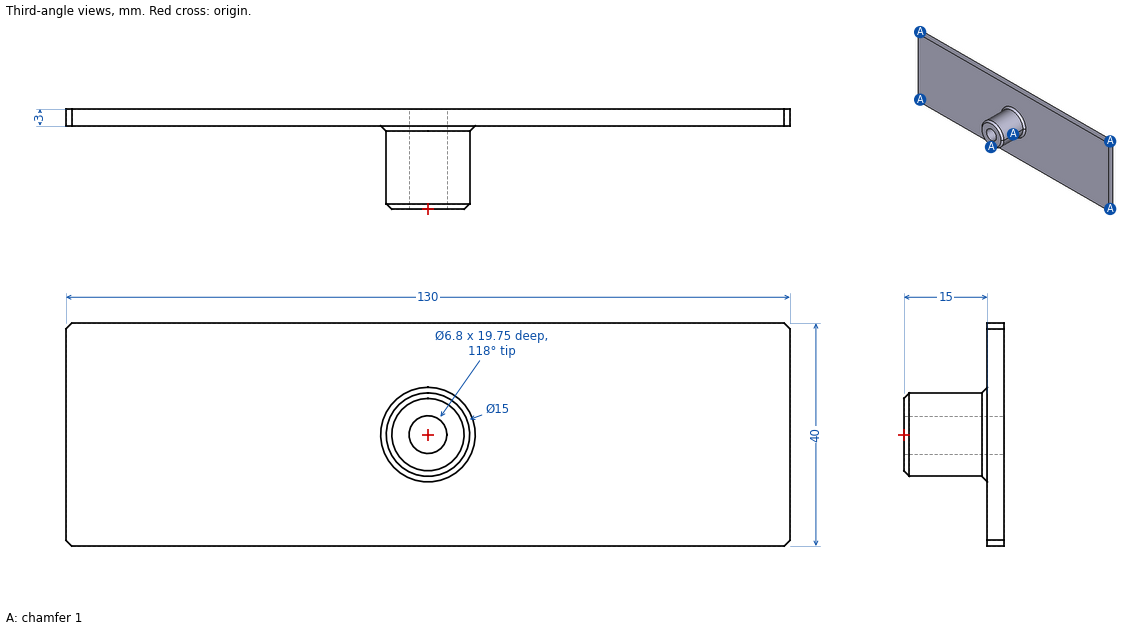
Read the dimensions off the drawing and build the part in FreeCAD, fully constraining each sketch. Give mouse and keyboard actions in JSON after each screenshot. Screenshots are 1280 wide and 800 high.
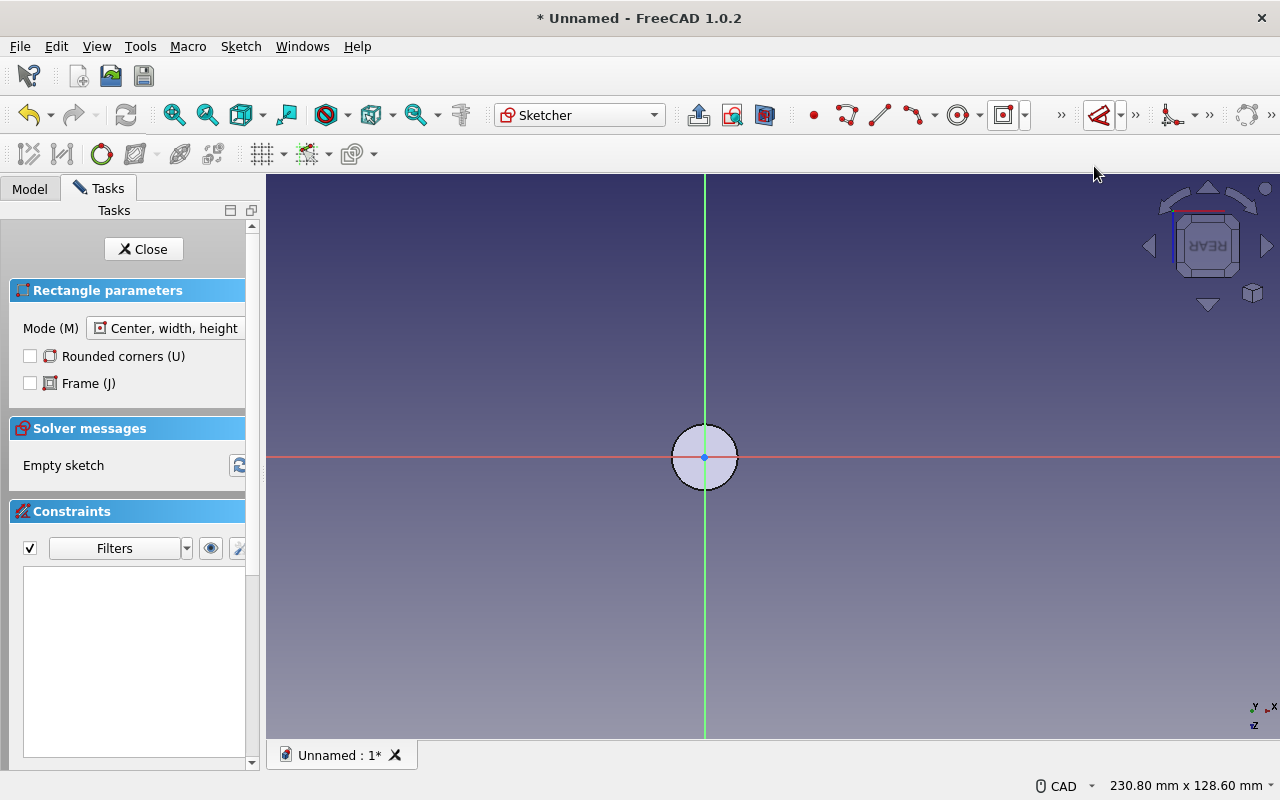
{"action": "left_click", "coordinate": [705, 457]}
{"action": "mouse_move", "coordinate": [990, 369]}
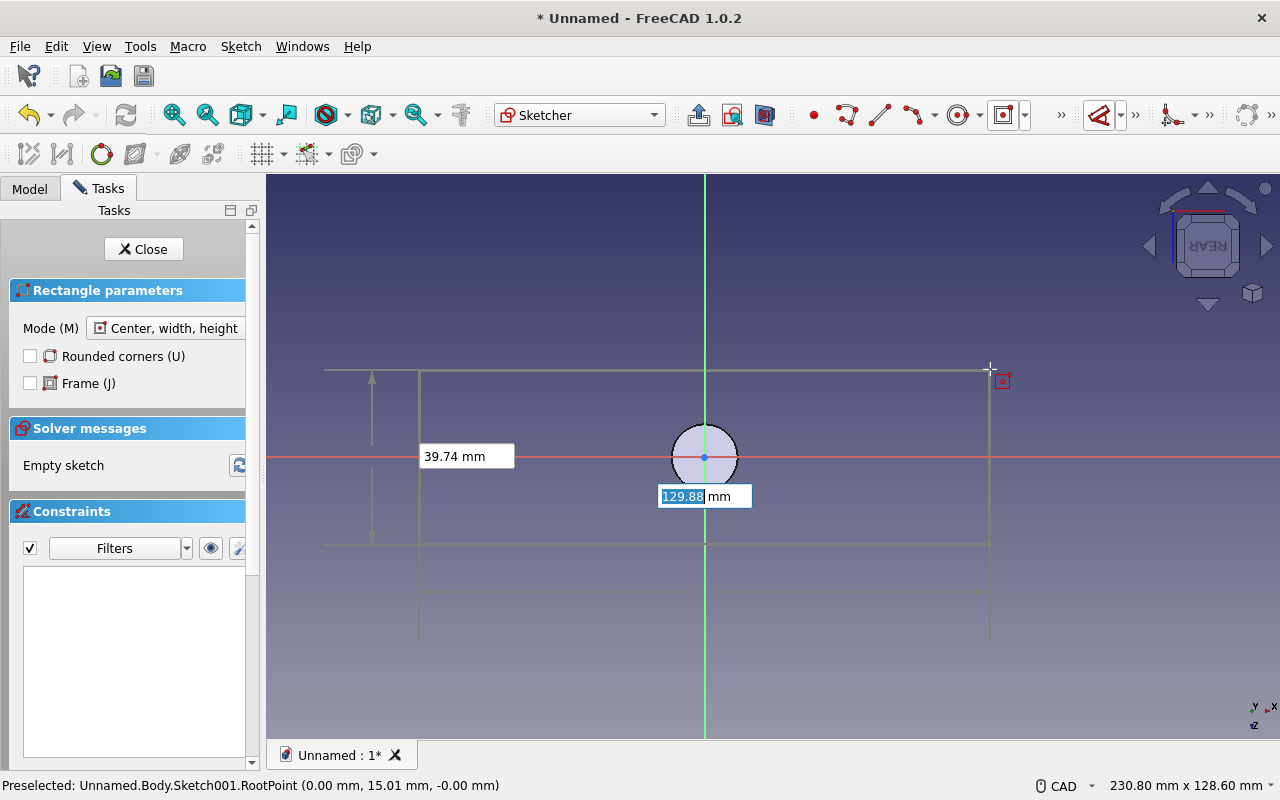
{"action": "type", "text": "130"}
{"action": "key", "text": "Tab"}
{"action": "type", "text": "40"}
{"action": "key", "text": "Return"}
{"action": "key", "text": "Escape"}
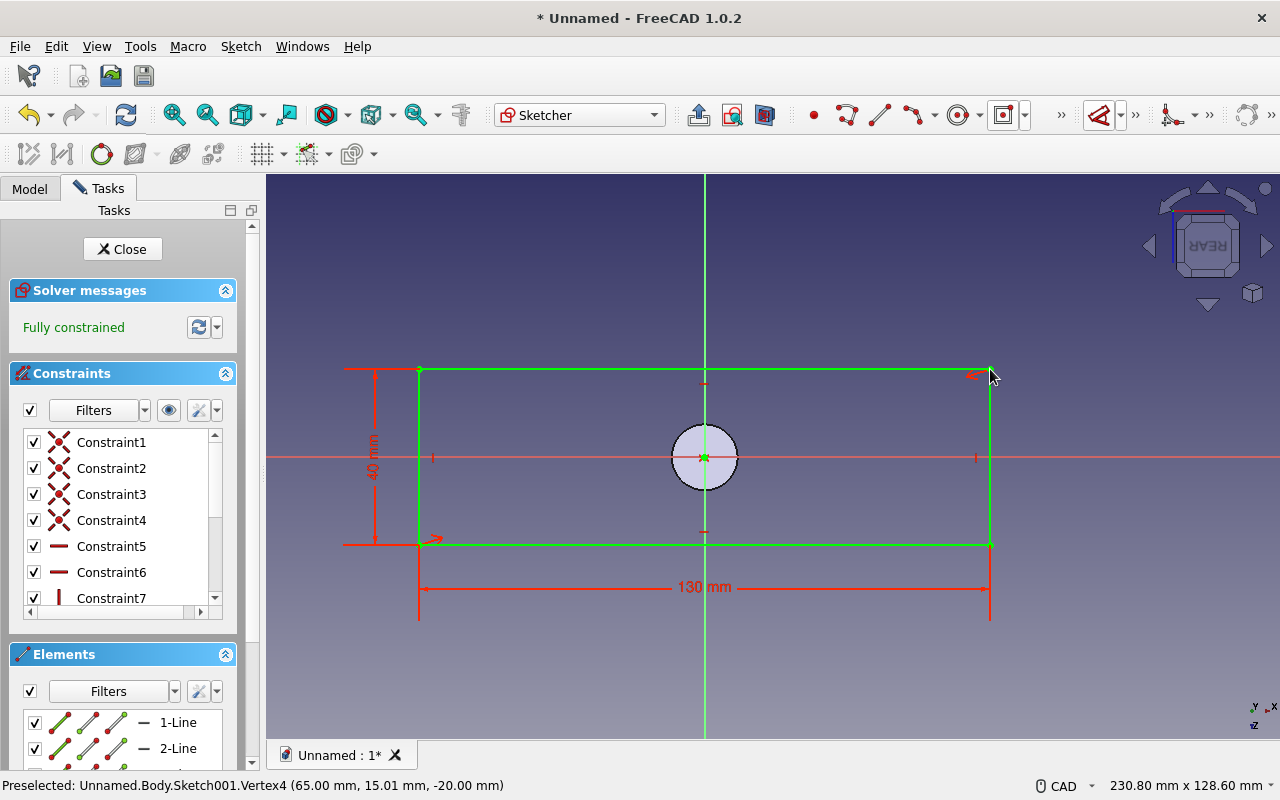
{"action": "left_click", "coordinate": [123, 249]}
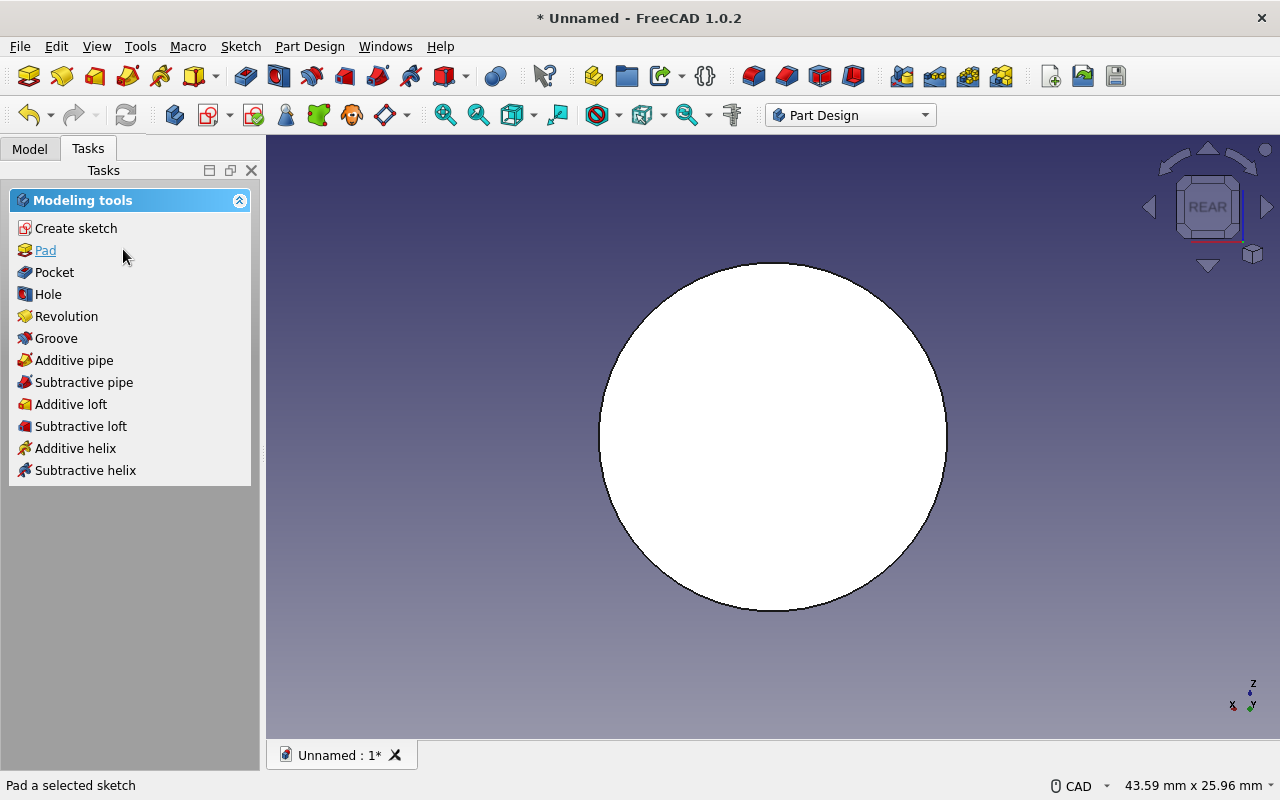
{"action": "left_click", "coordinate": [29, 76]}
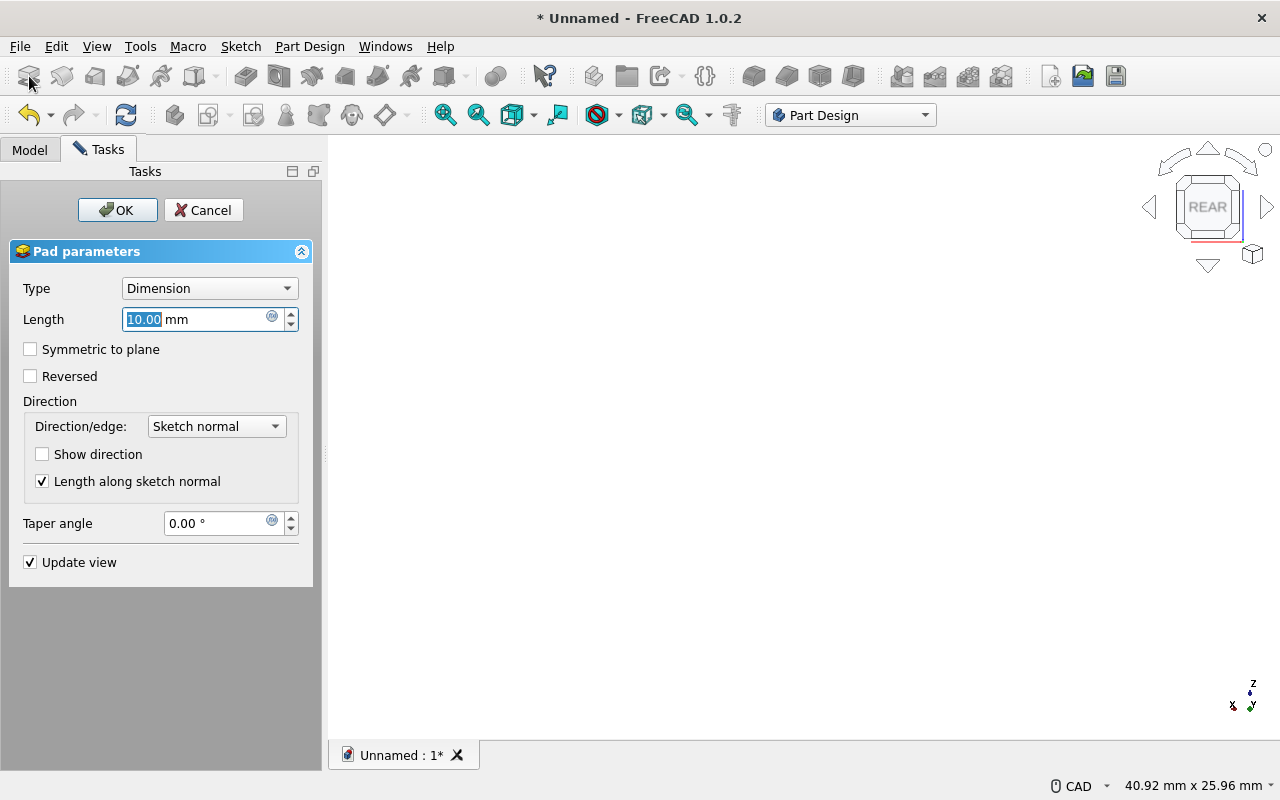
{"action": "type", "text": "3"}
{"action": "key", "text": "Tab"}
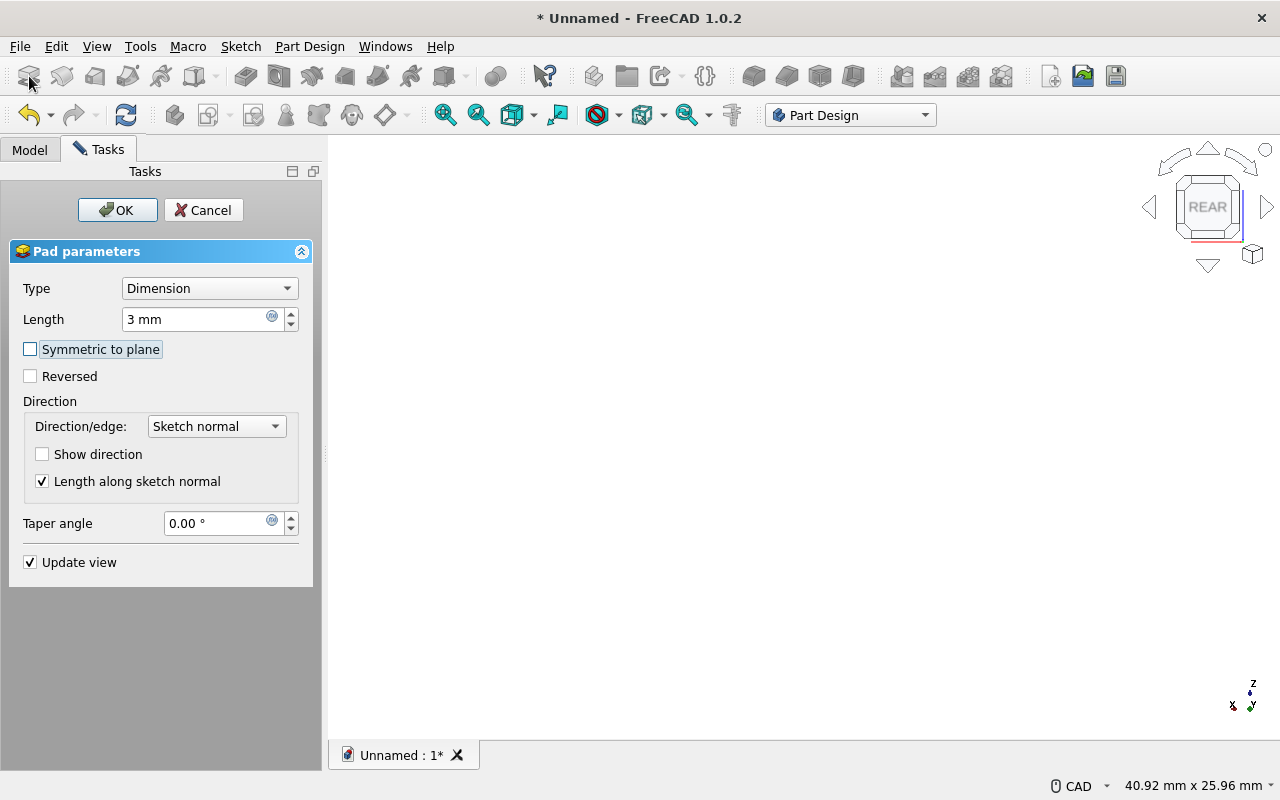
{"action": "left_click", "coordinate": [118, 210]}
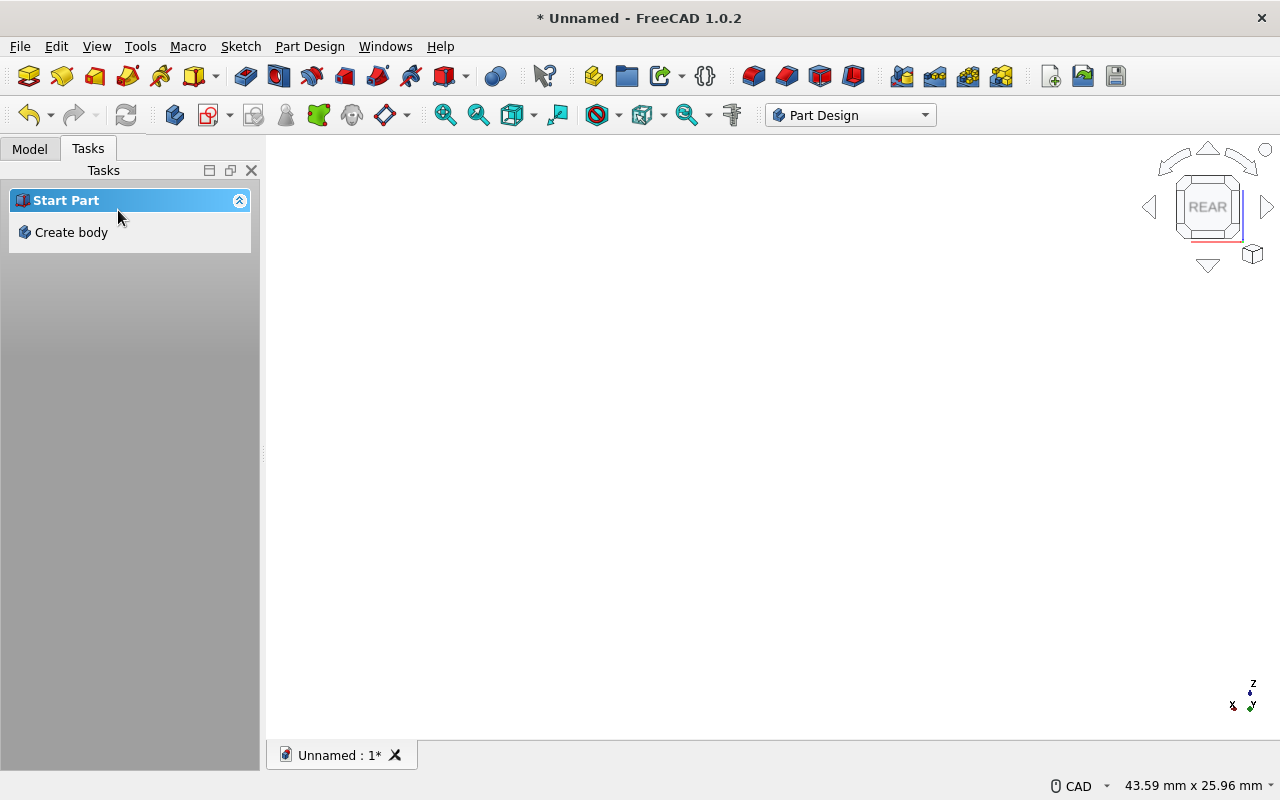
{"action": "left_click", "coordinate": [446, 116]}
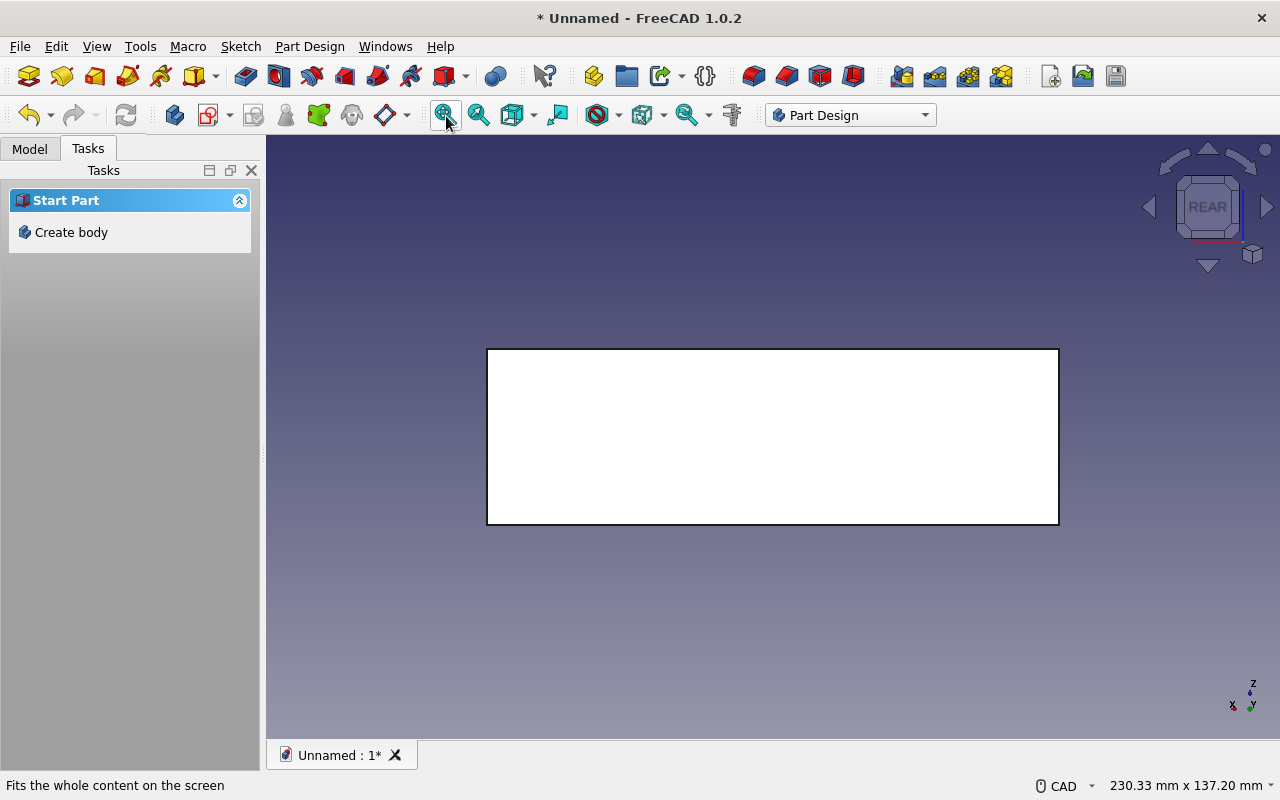
{"action": "left_click", "coordinate": [208, 116]}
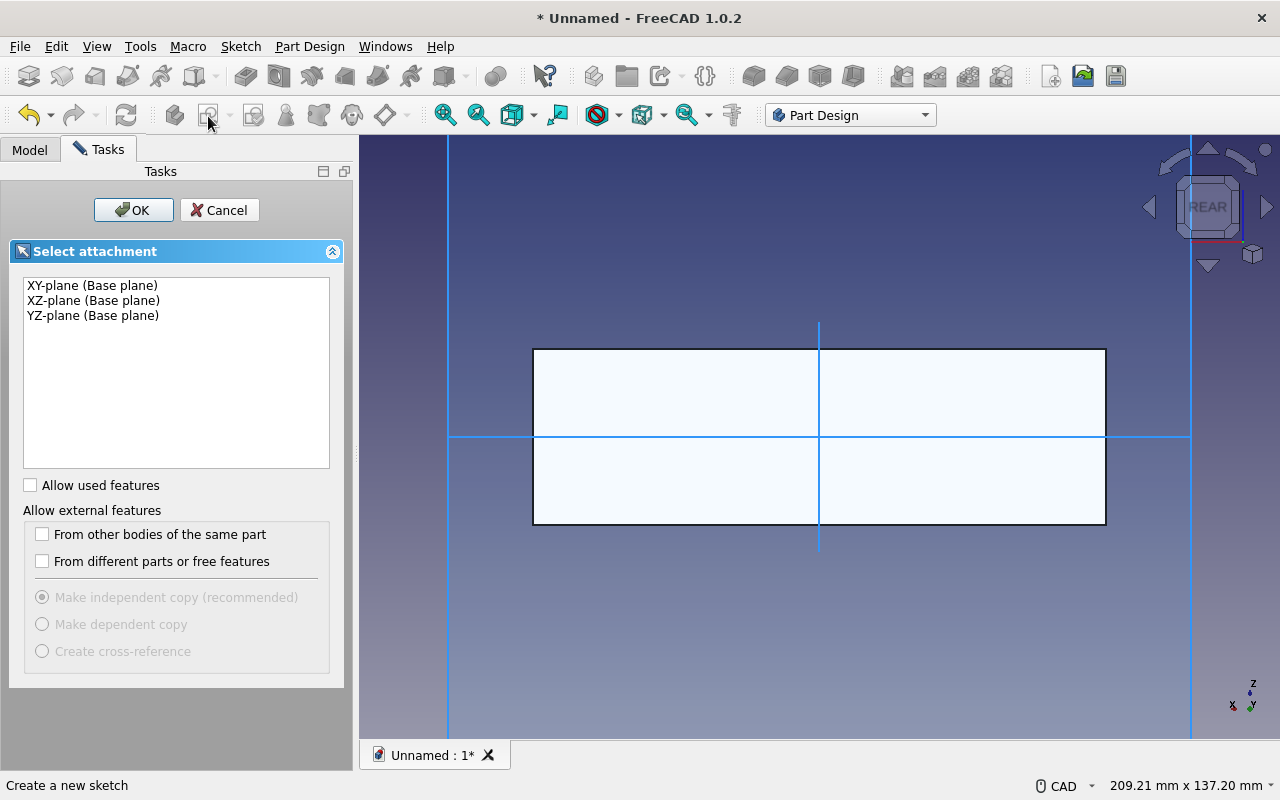
{"action": "left_click", "coordinate": [84, 300]}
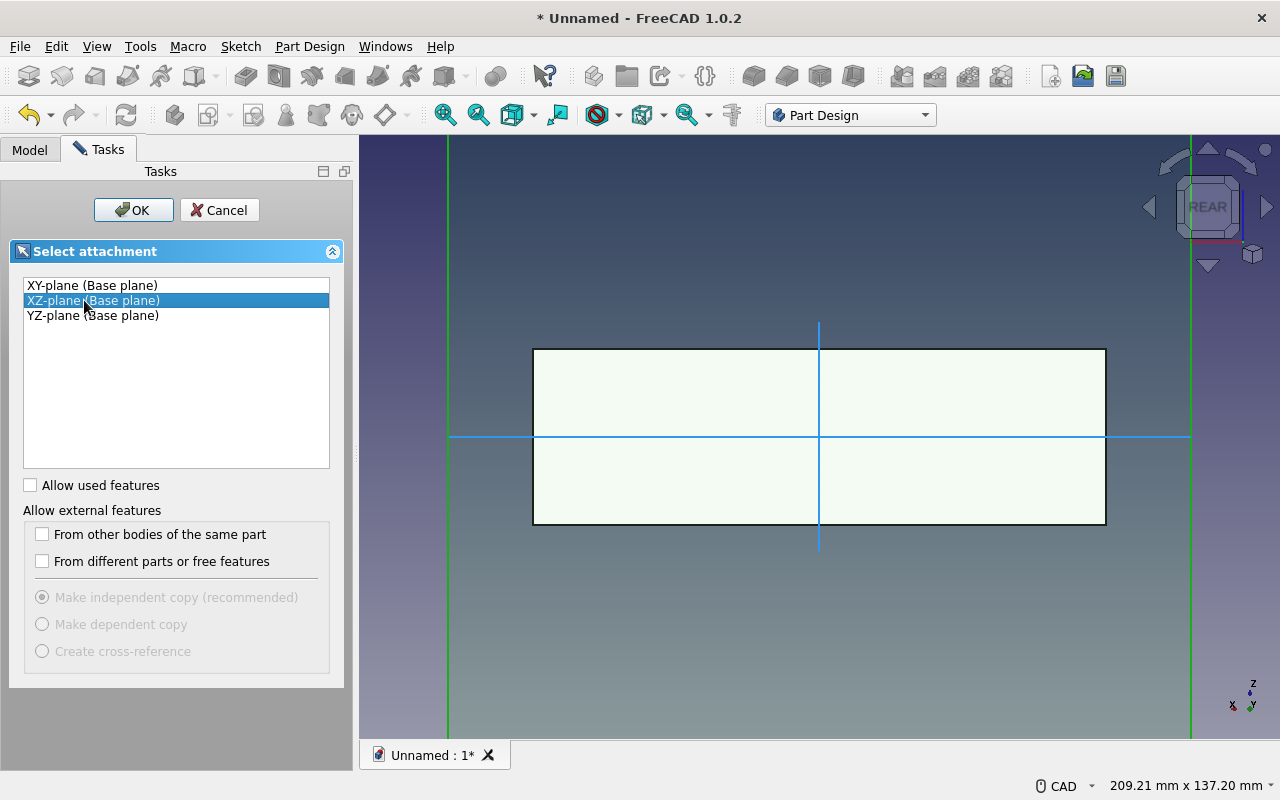
{"action": "left_click", "coordinate": [134, 210]}